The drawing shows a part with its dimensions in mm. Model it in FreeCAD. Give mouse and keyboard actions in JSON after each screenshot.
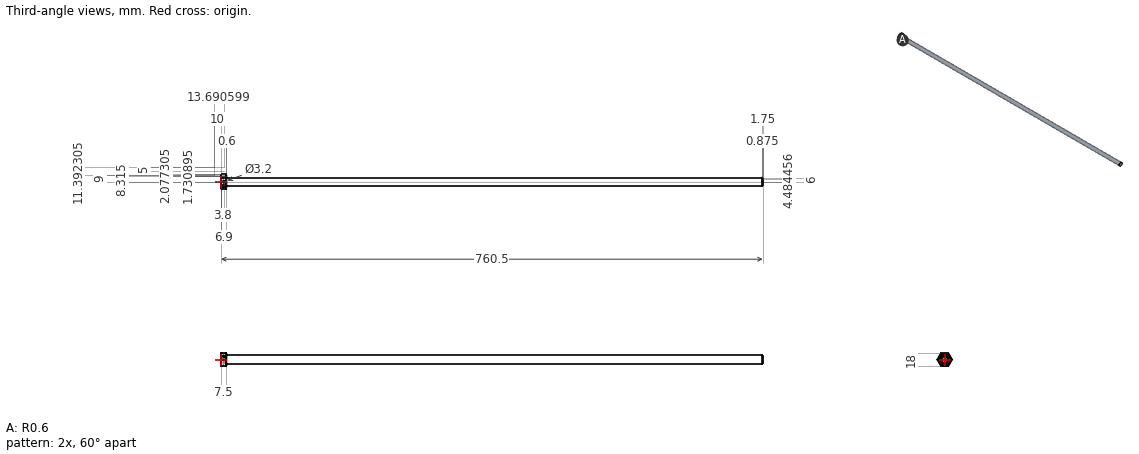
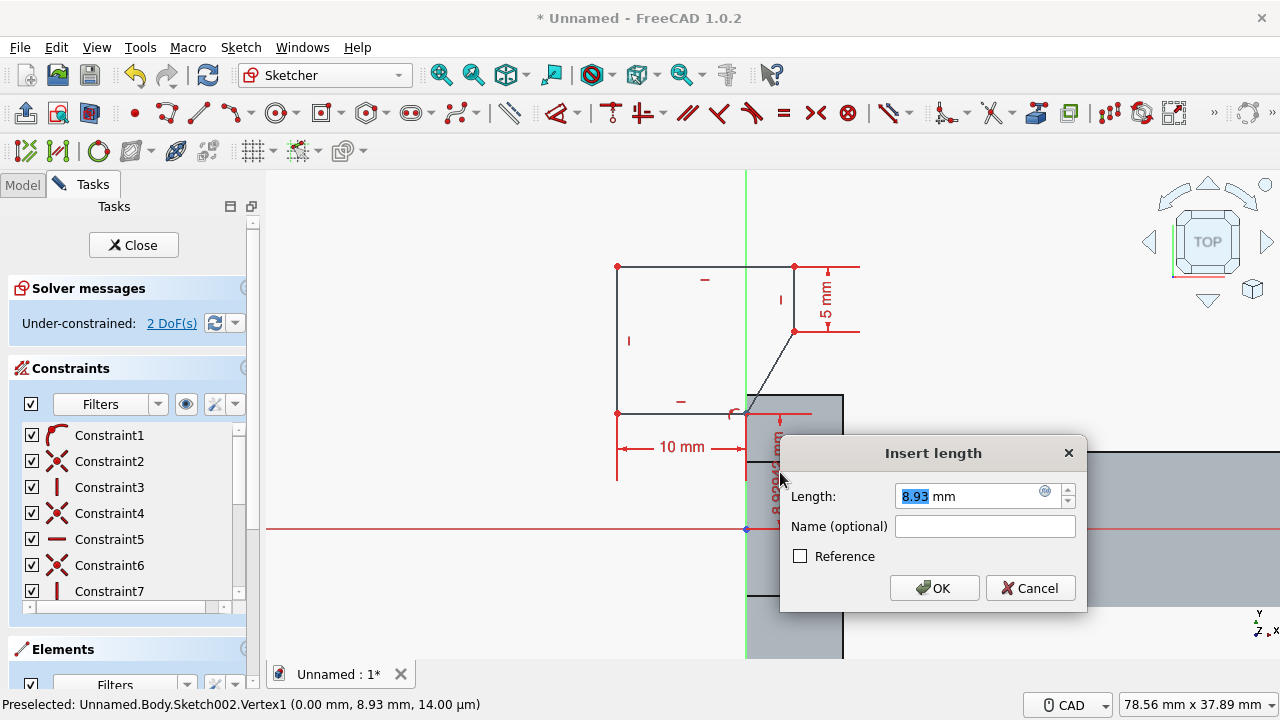
{"action": "type", "text": "9"}
{"action": "key", "text": "Return"}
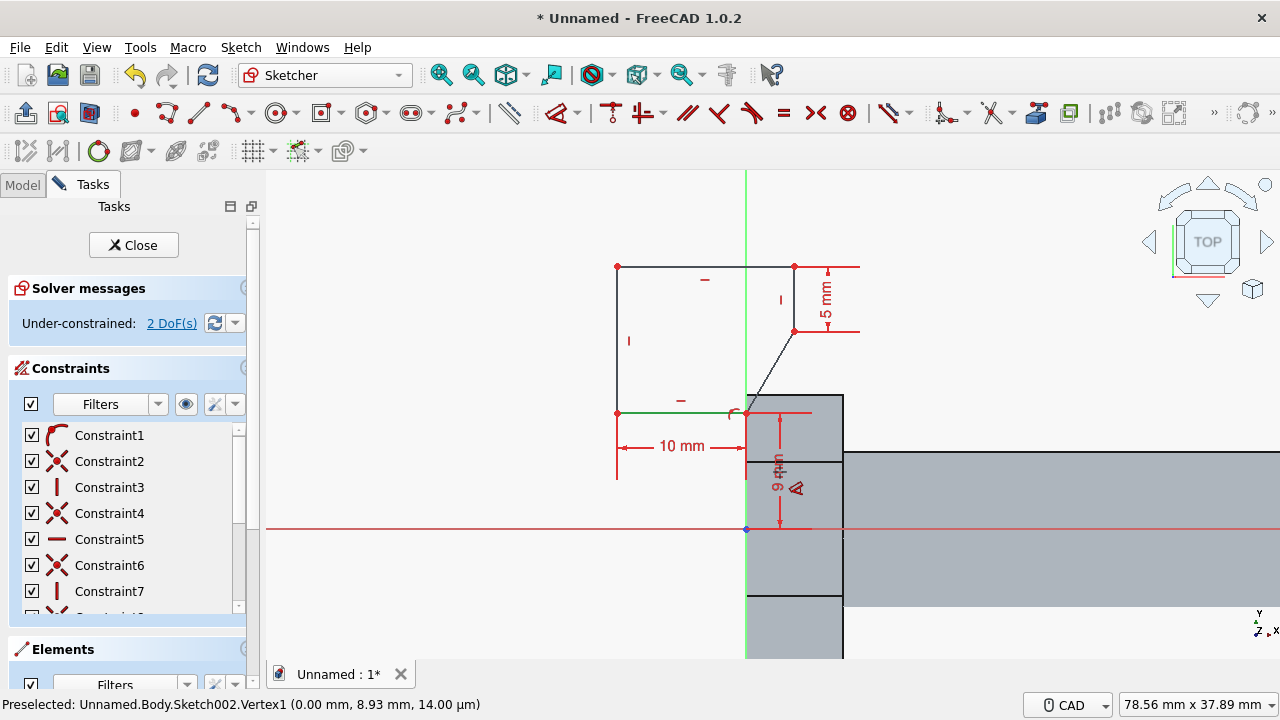
{"action": "left_click", "coordinate": [670, 267]}
{"action": "left_click", "coordinate": [706, 233]}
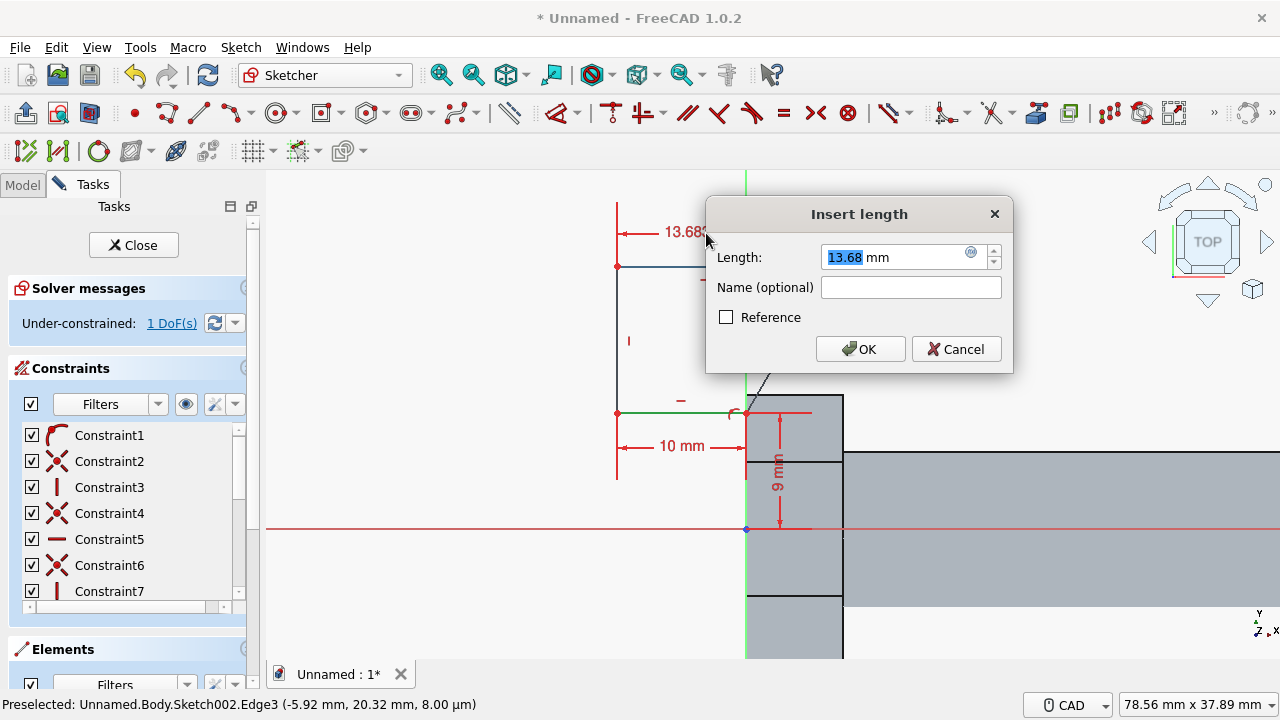
{"action": "type", "text": "13.690599"}
{"action": "key", "text": "Return"}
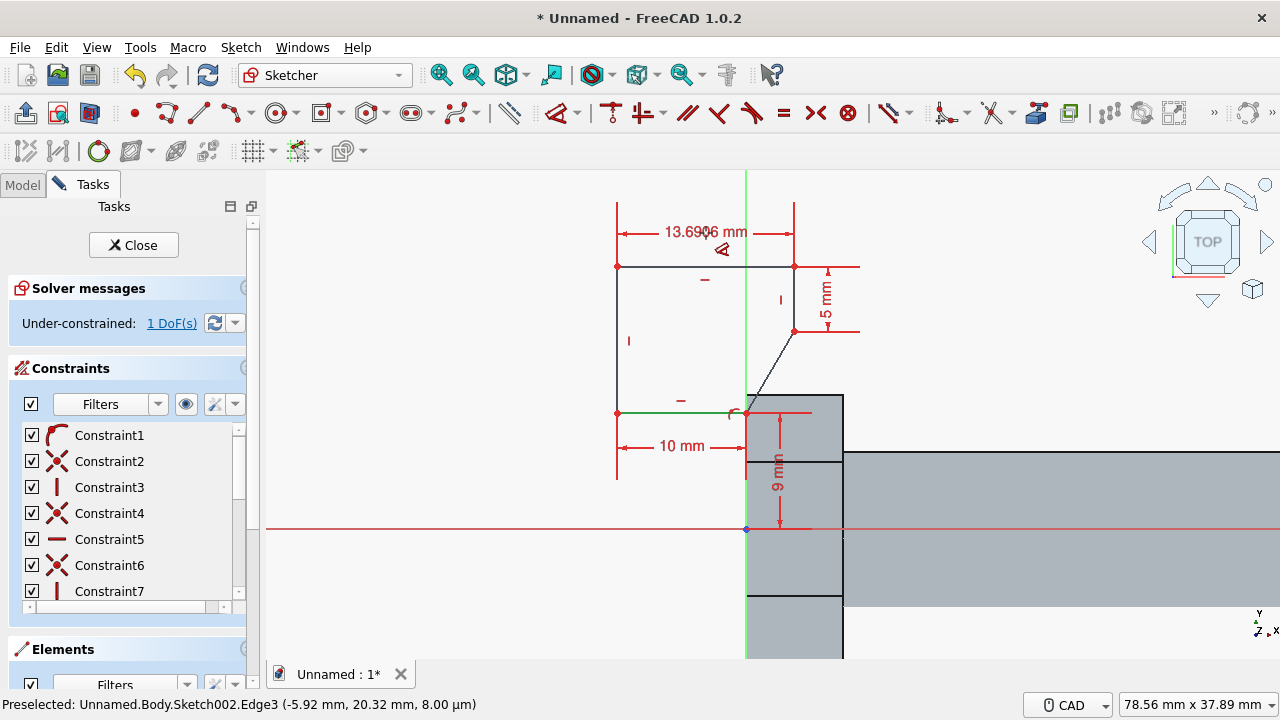
{"action": "left_click", "coordinate": [617, 311]}
{"action": "left_click", "coordinate": [583, 340]}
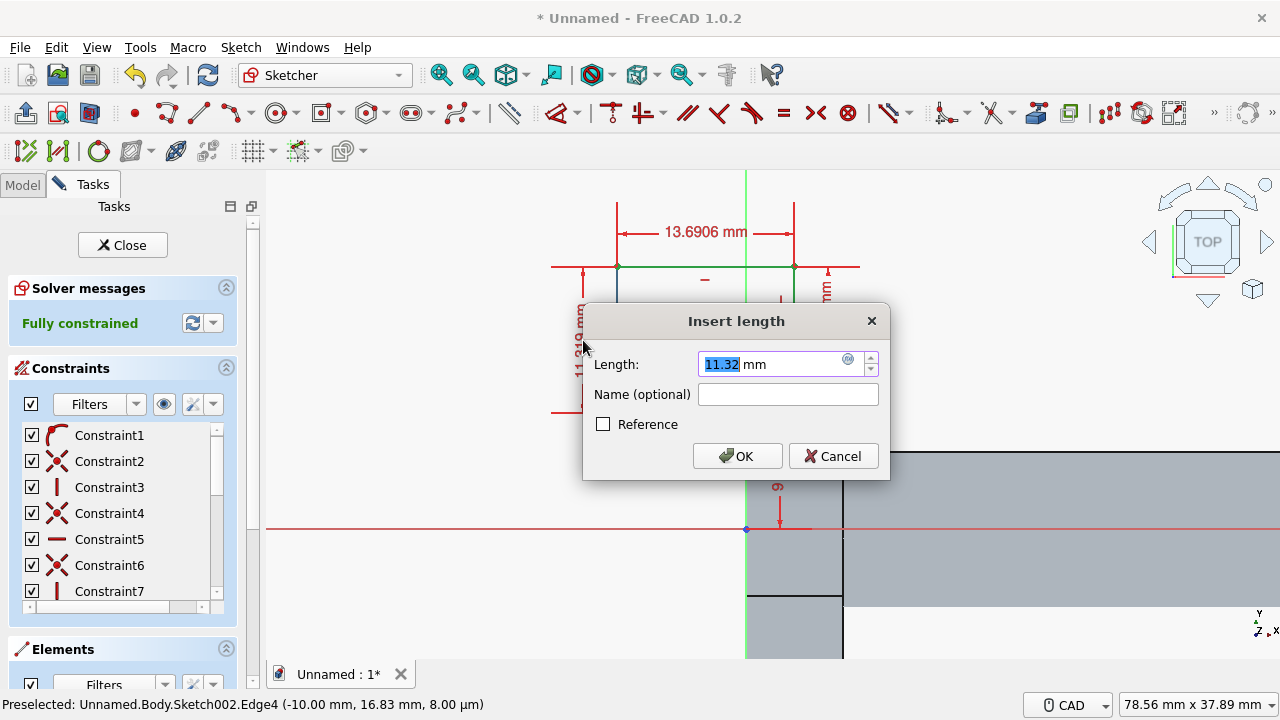
{"action": "type", "text": "11.392305"}
{"action": "key", "text": "Return"}
{"action": "key", "text": "Escape"}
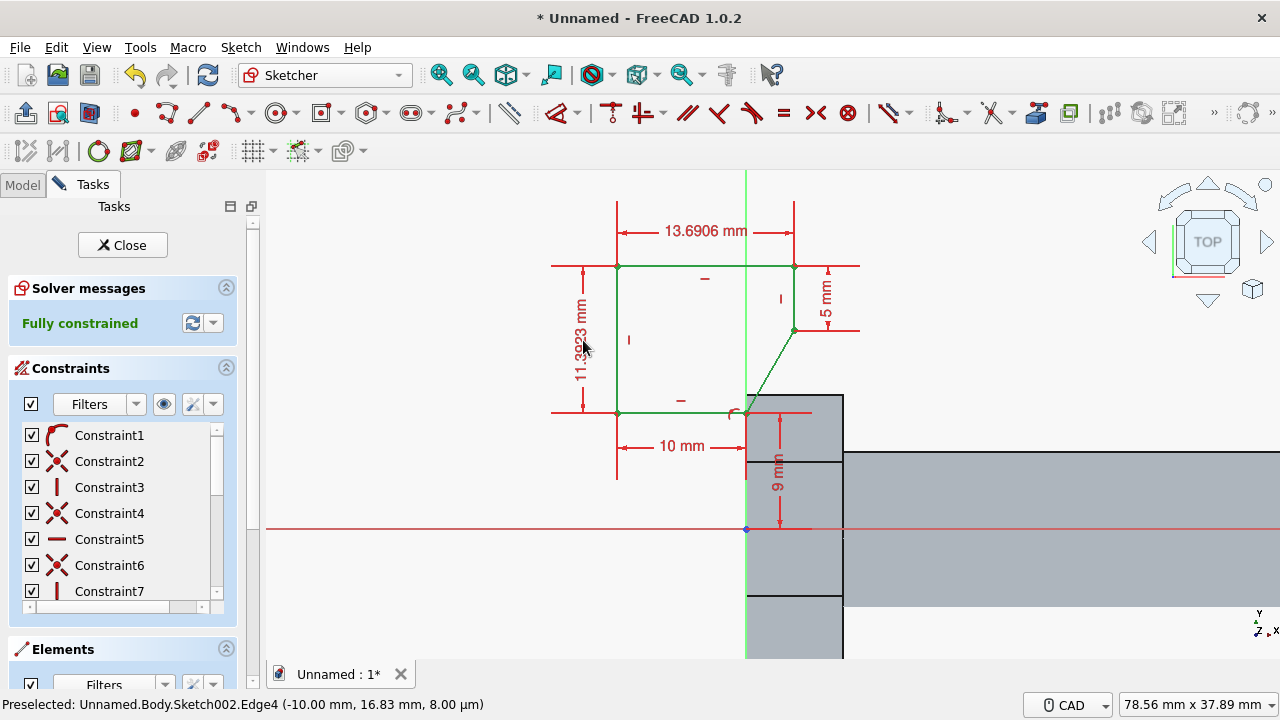
{"action": "left_click", "coordinate": [123, 245]}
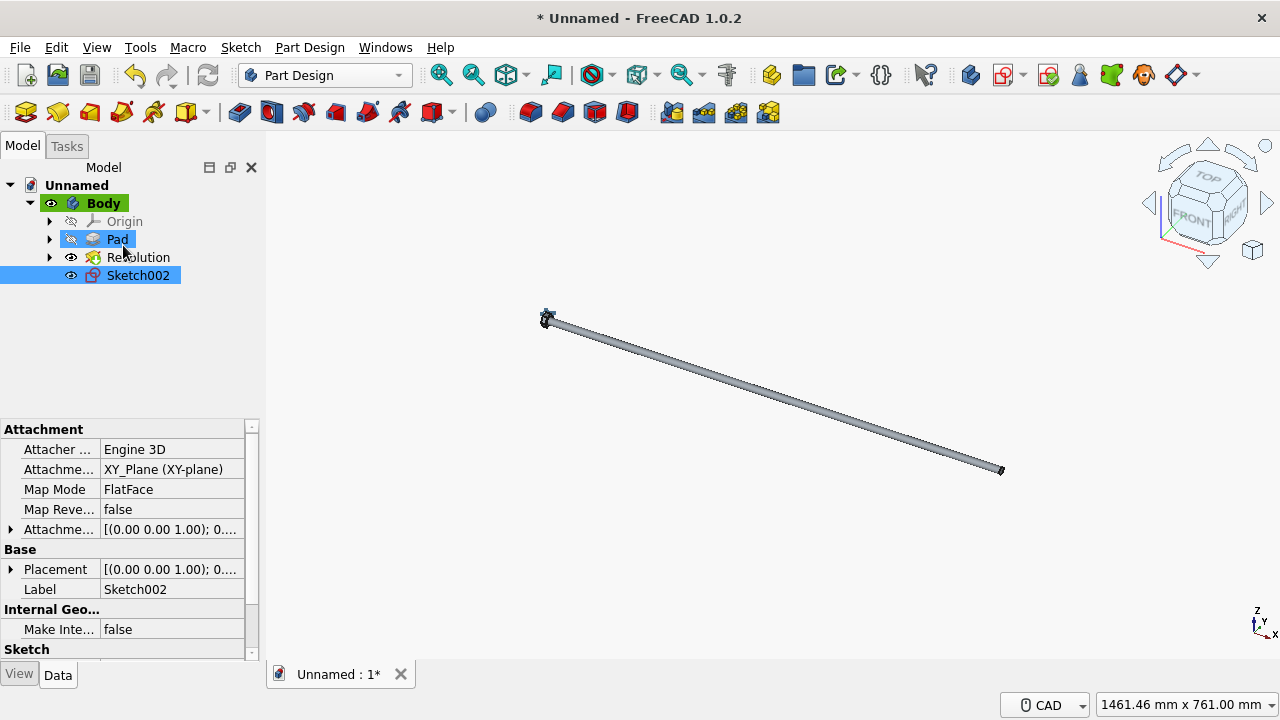
{"action": "left_click", "coordinate": [304, 112]}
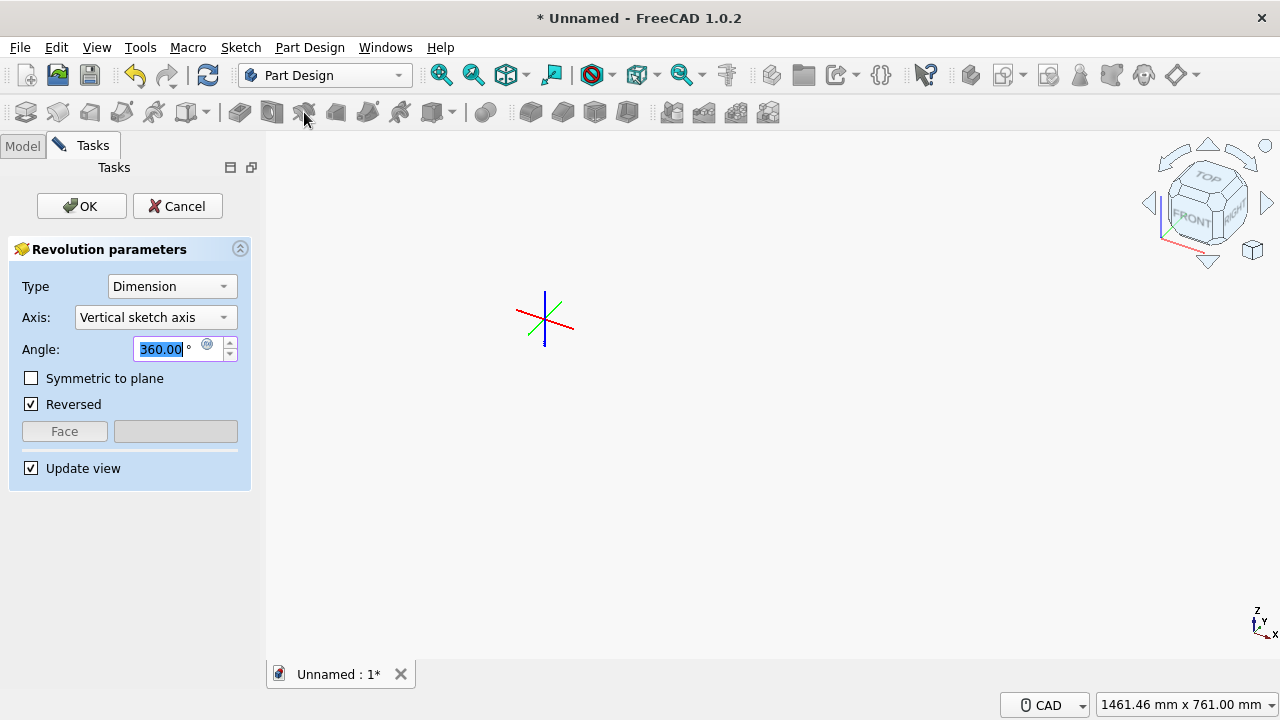
{"action": "left_click", "coordinate": [156, 318]}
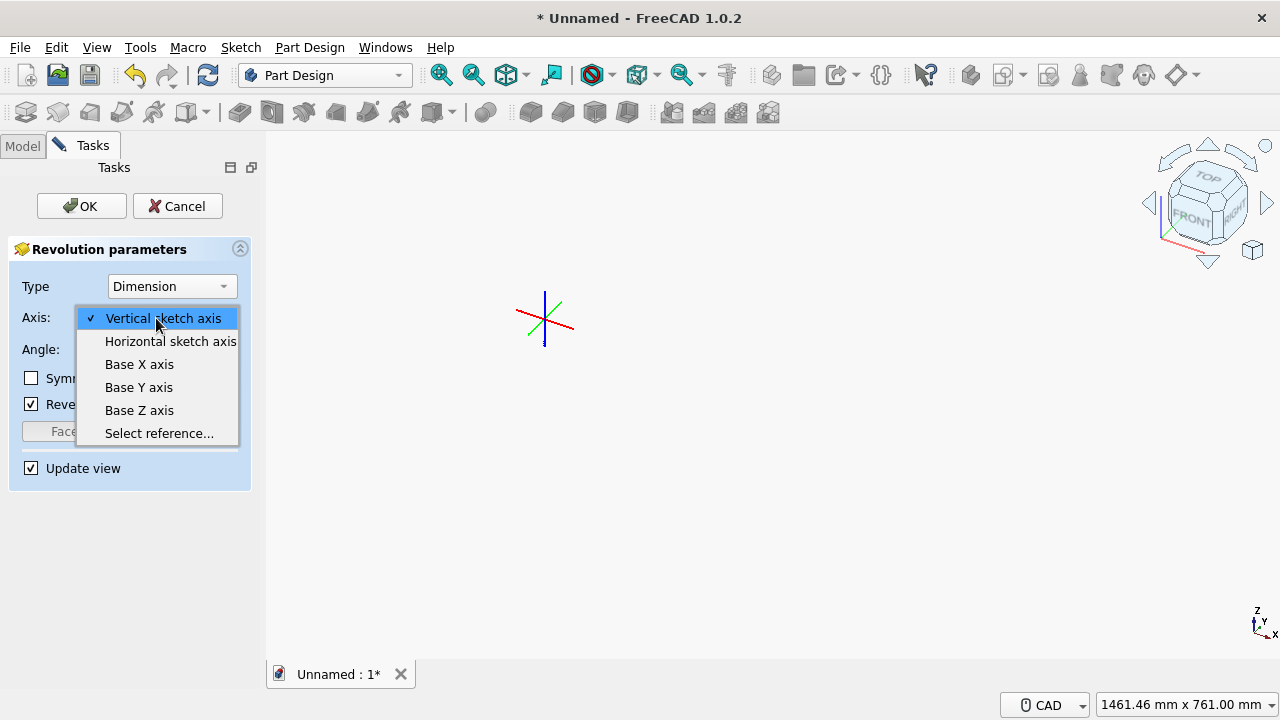
{"action": "left_click", "coordinate": [156, 342]}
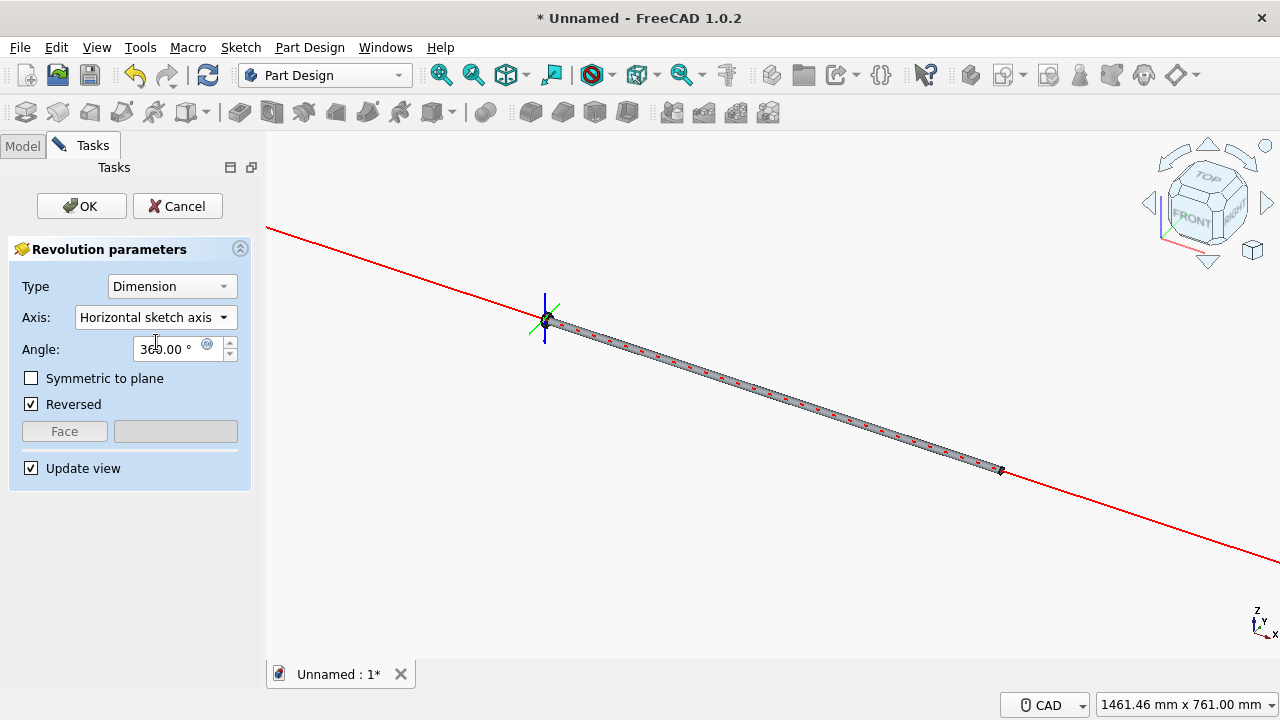
{"action": "left_click", "coordinate": [82, 206]}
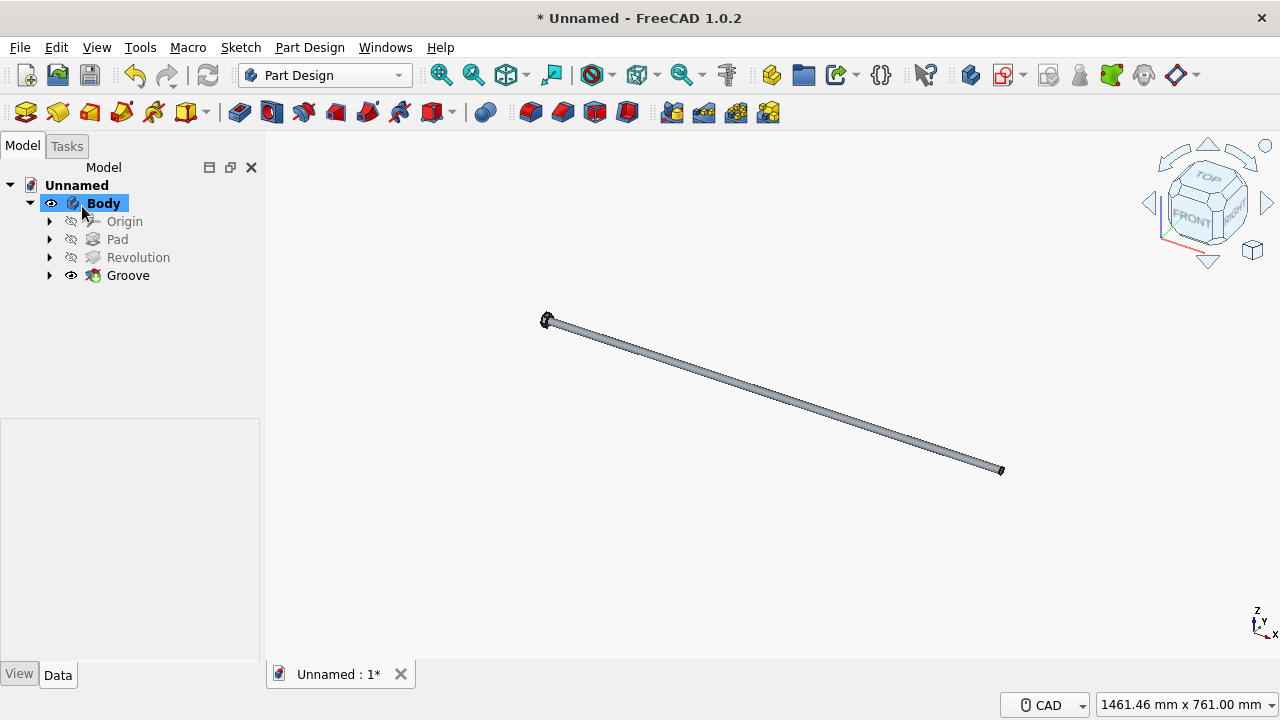
{"action": "left_click", "coordinate": [1004, 76]}